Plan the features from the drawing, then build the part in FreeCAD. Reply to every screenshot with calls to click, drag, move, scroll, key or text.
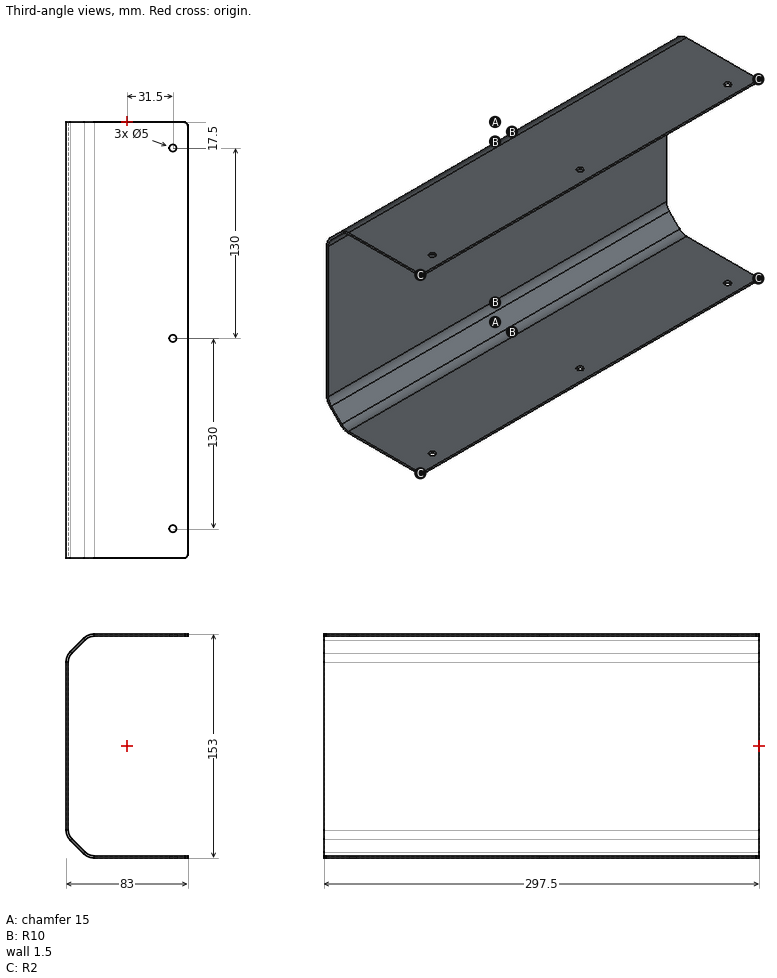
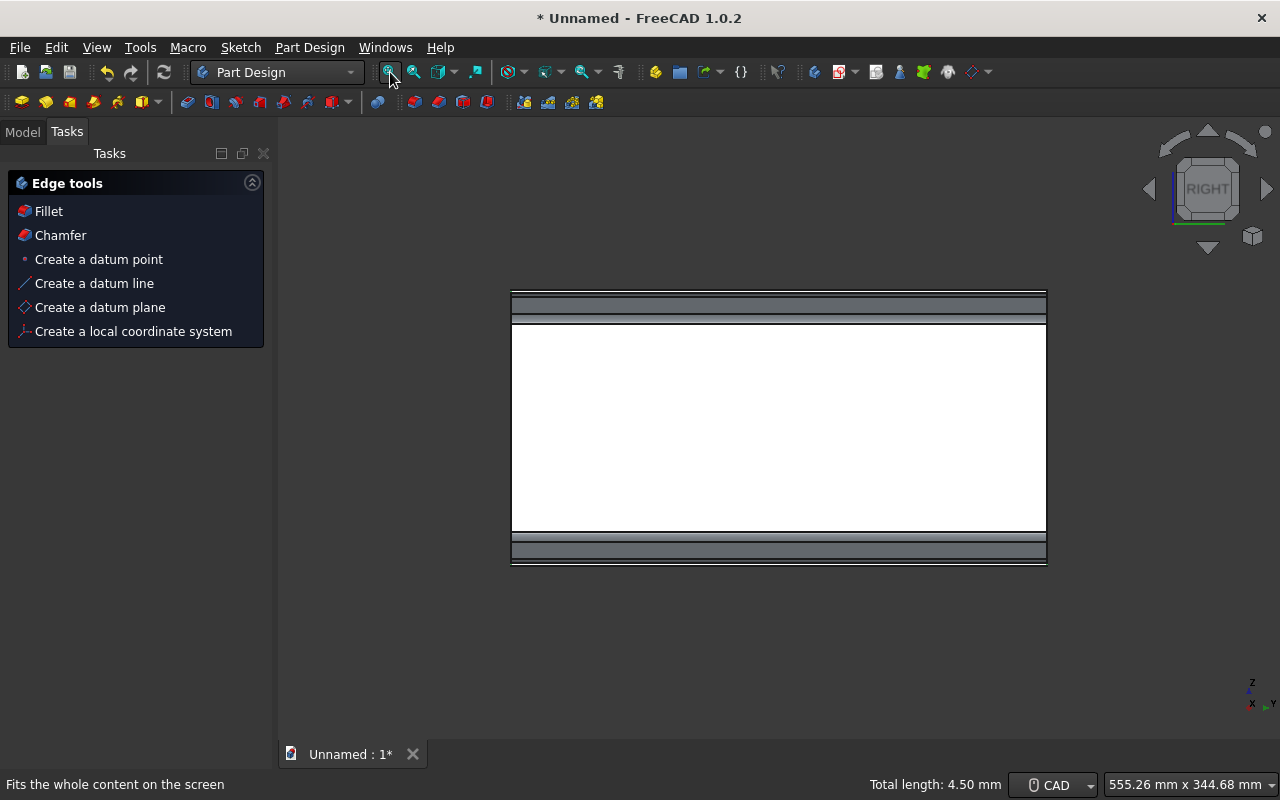
key(5)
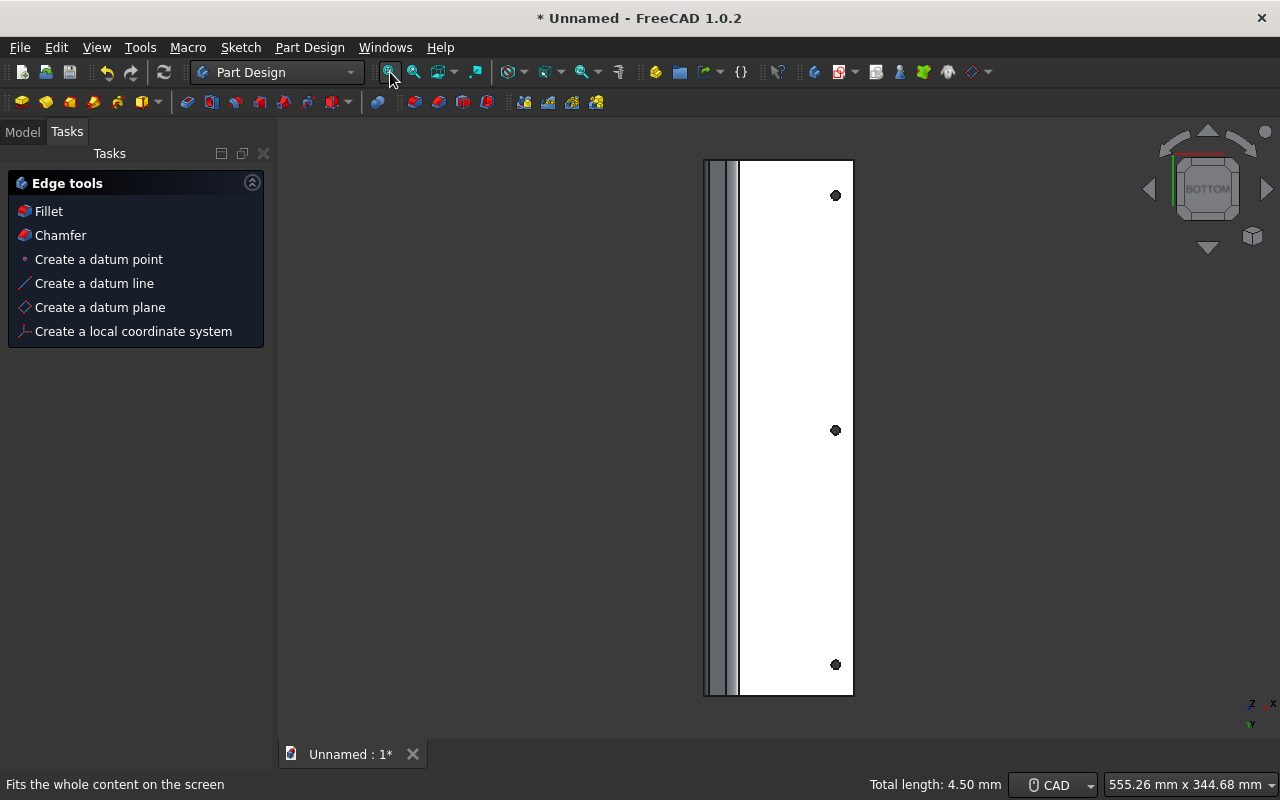
scroll(854, 695, up, 14)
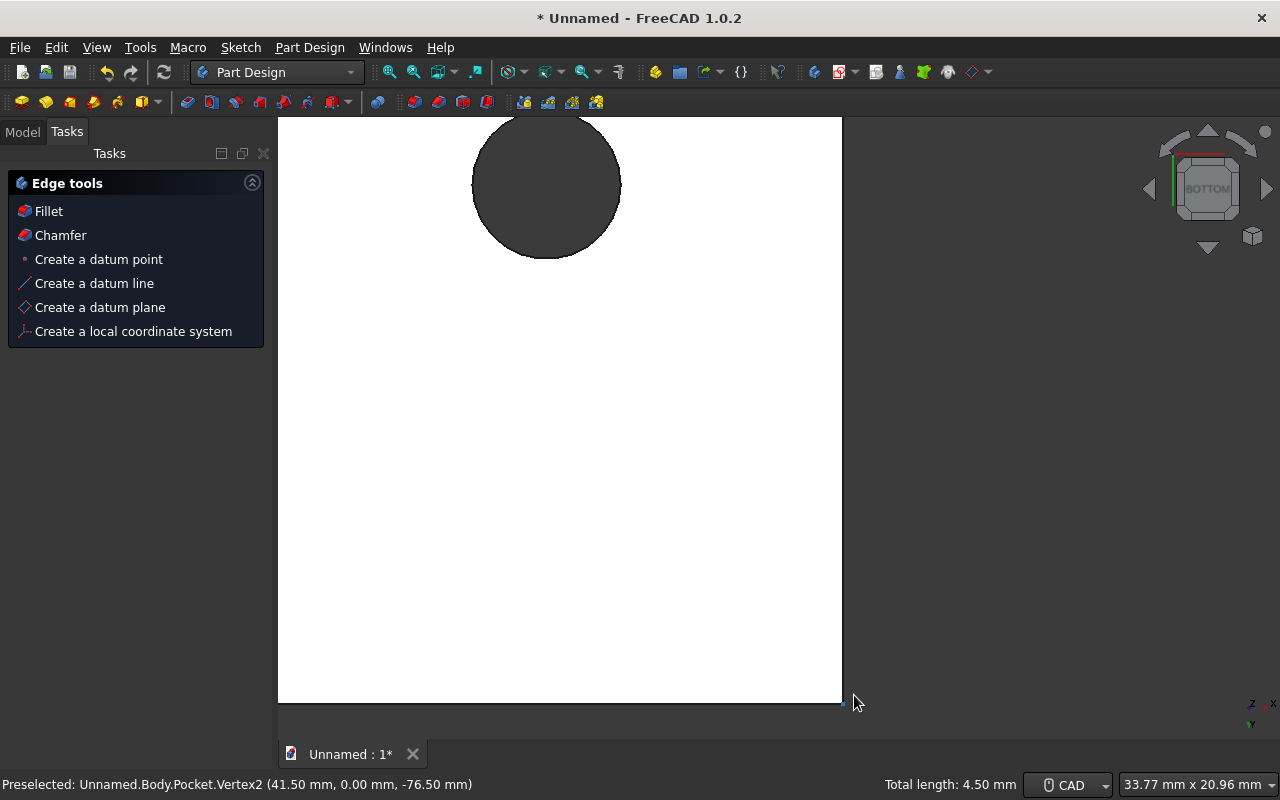
key(v)
key(f)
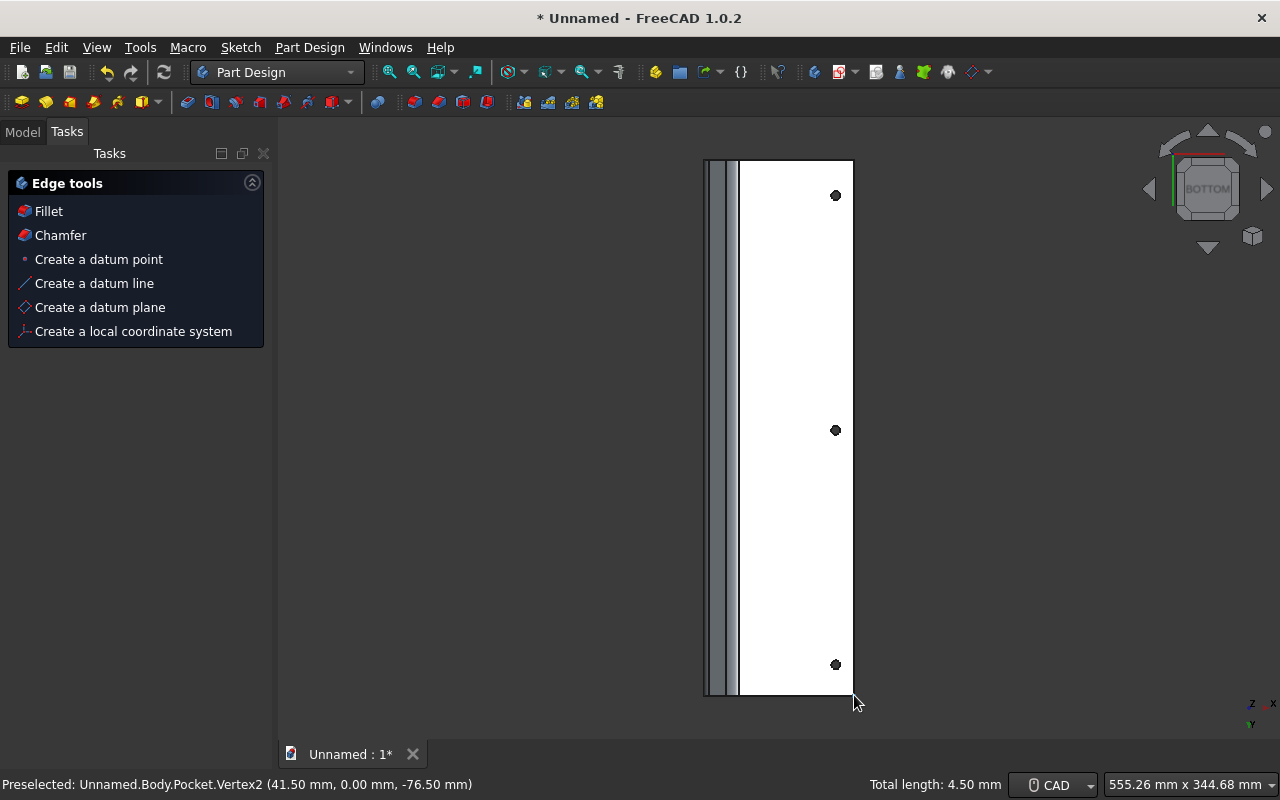
key(4)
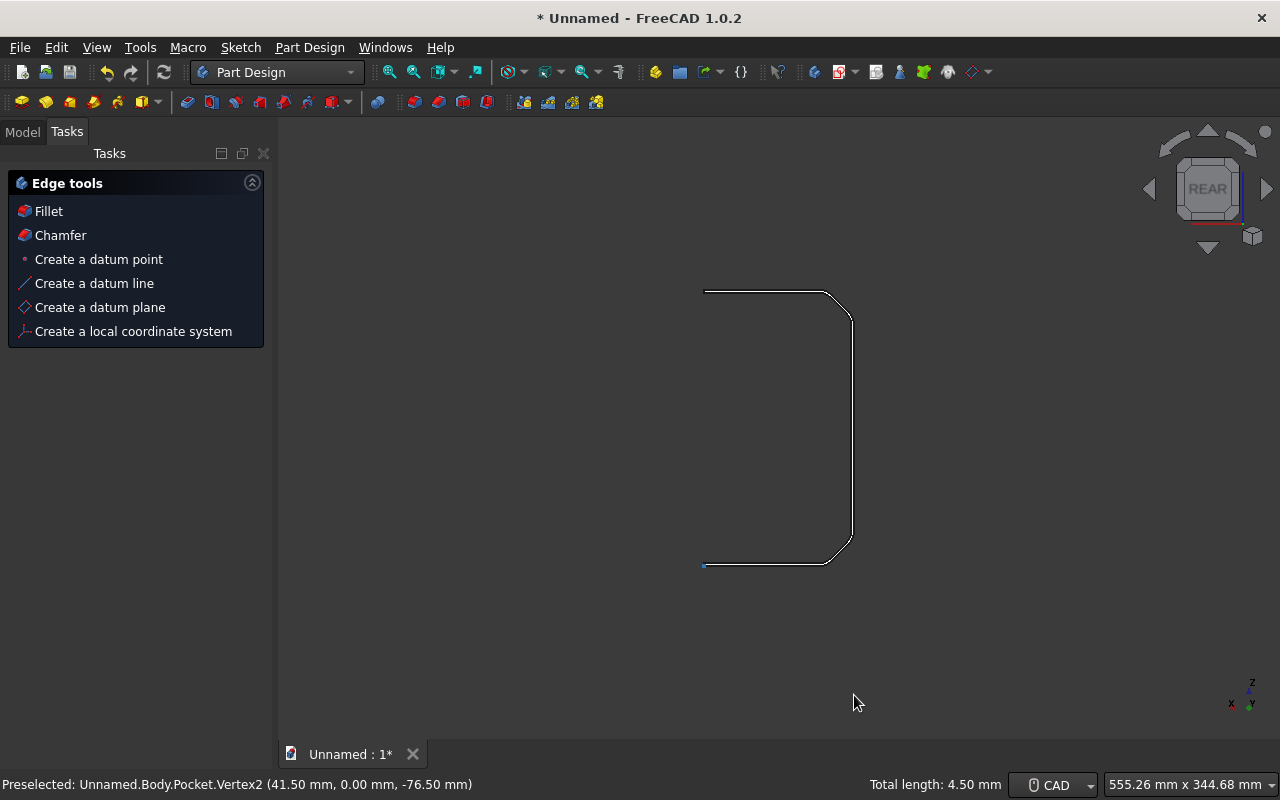
key(v)
key(f)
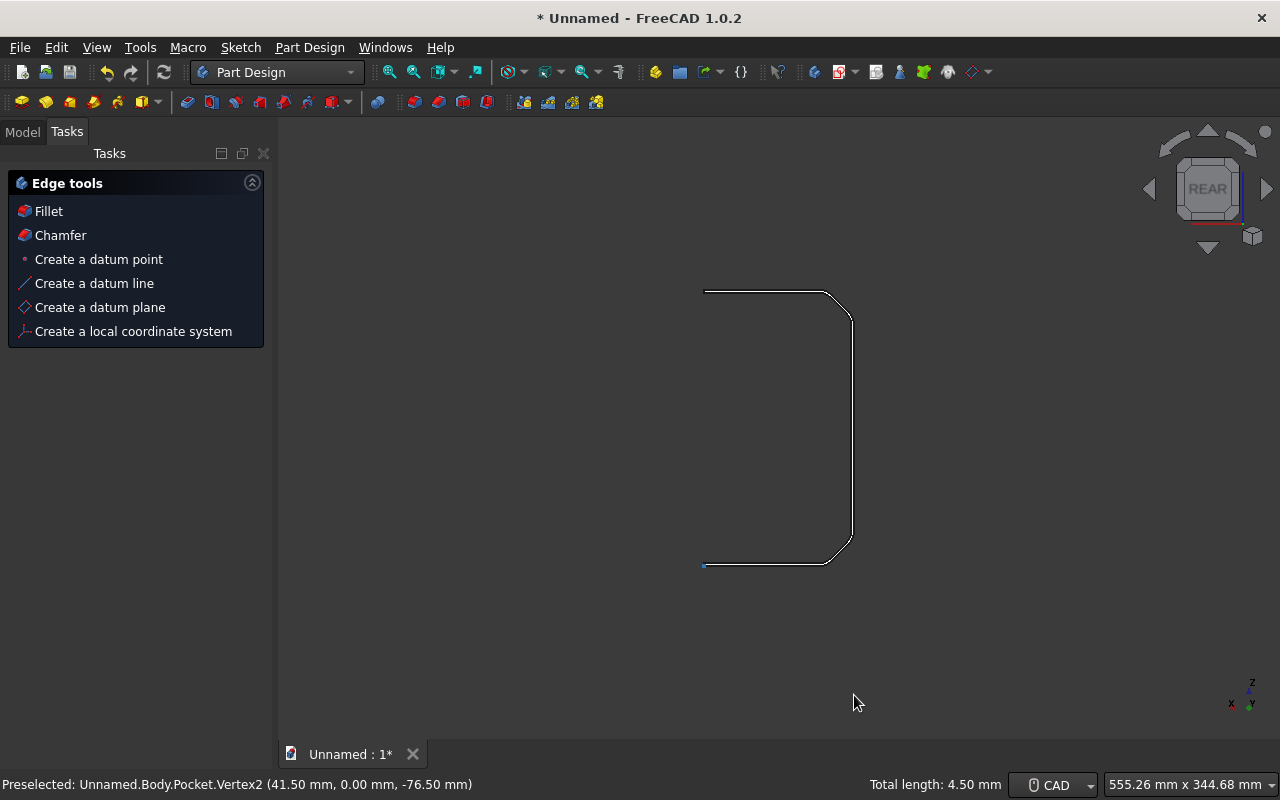
scroll(704, 290, up, 14)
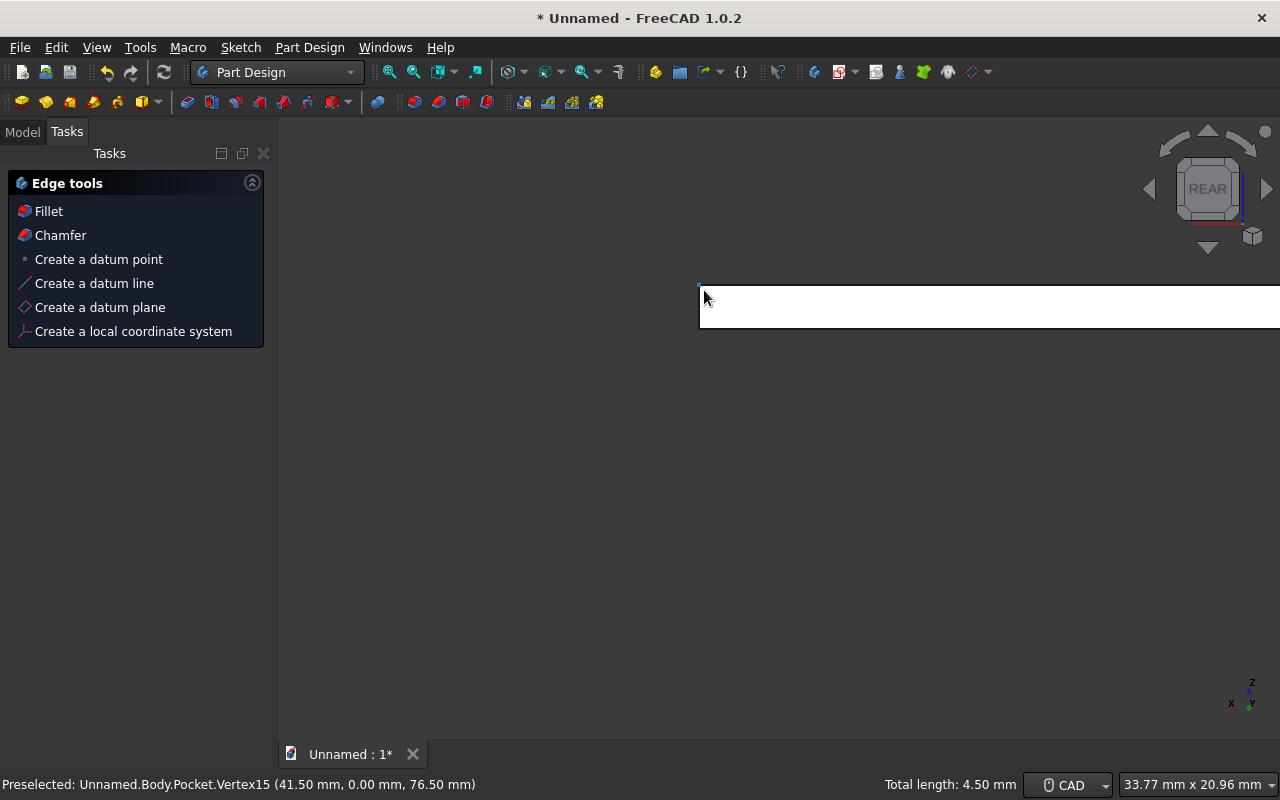
click(699, 306, ctrl)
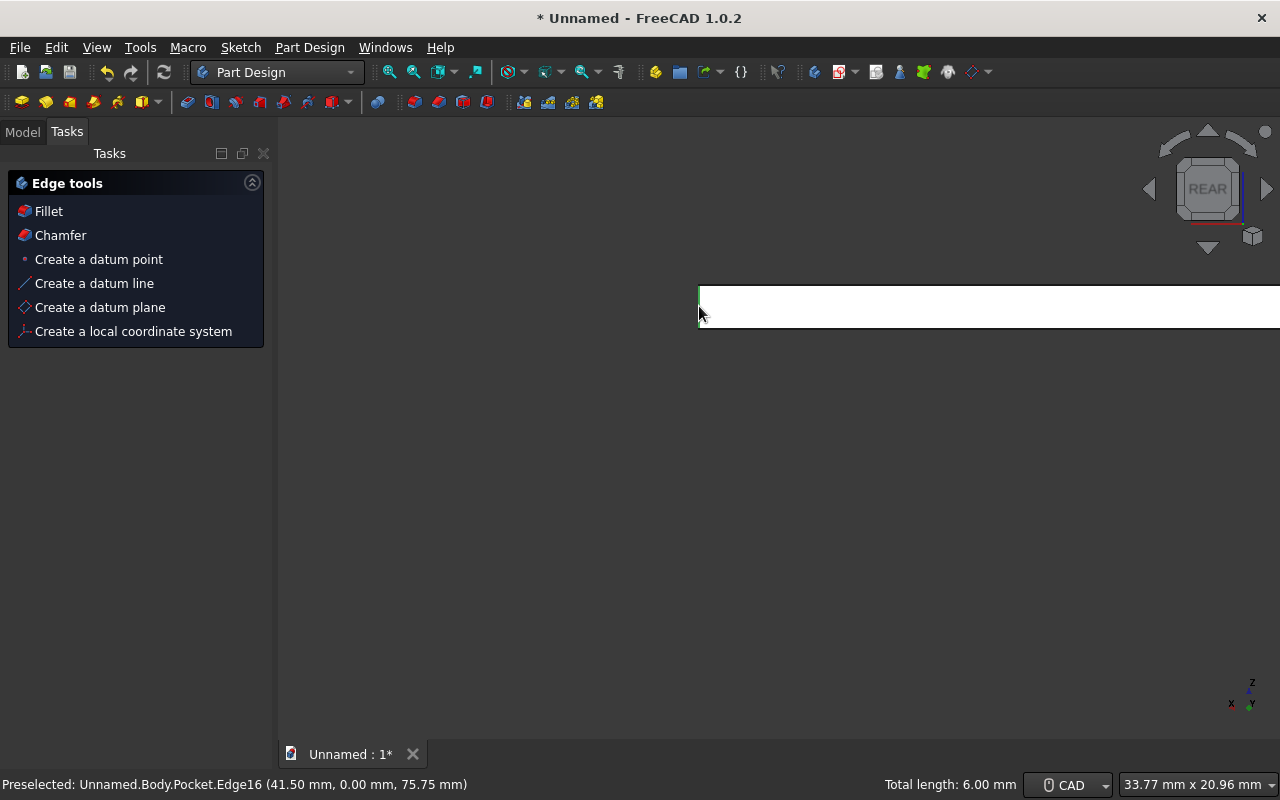
click(416, 102)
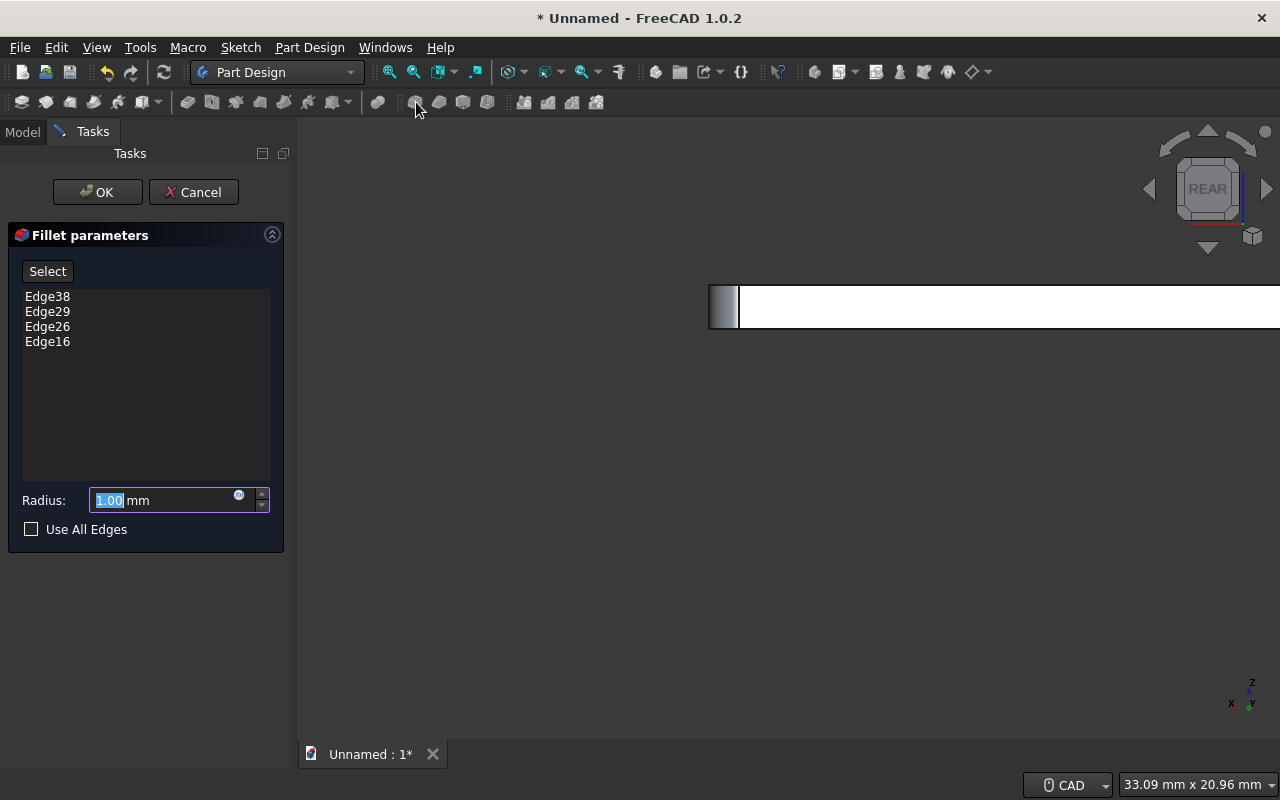
text(2)
key(Tab)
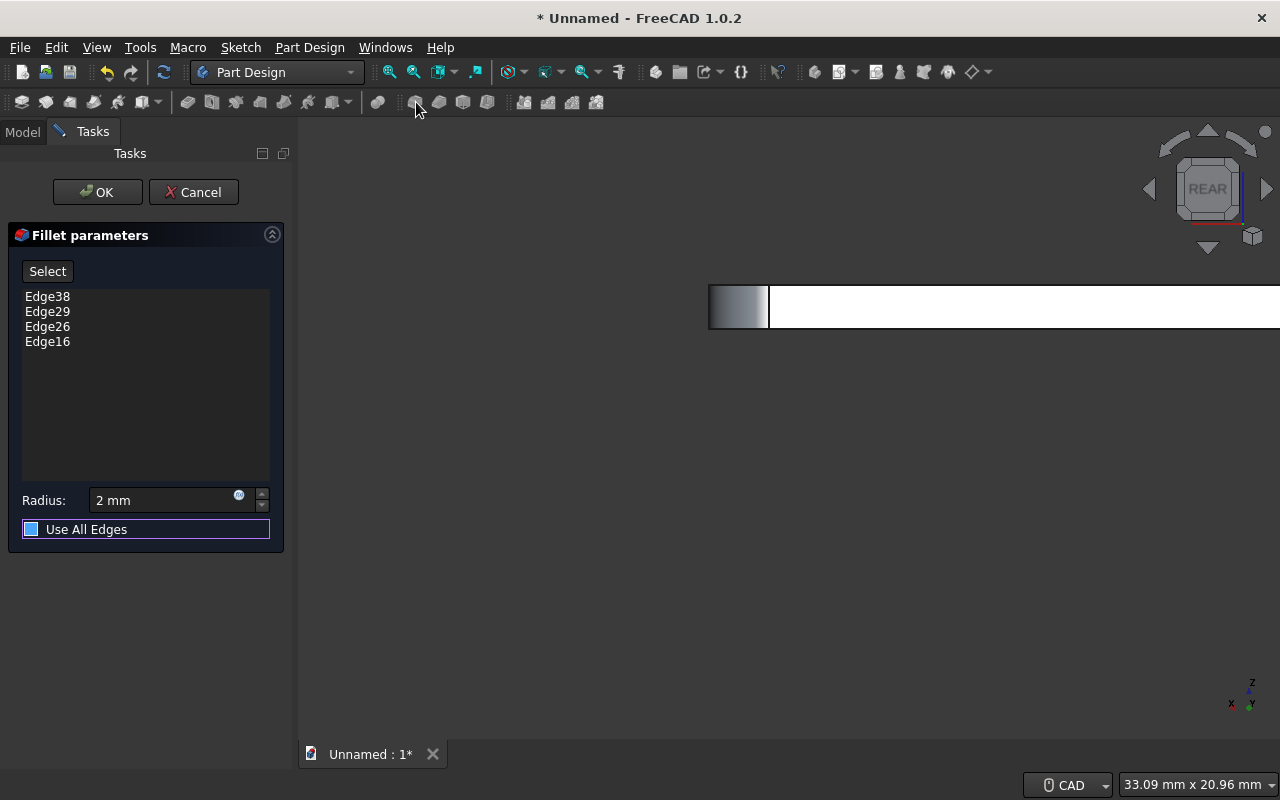
click(98, 192)